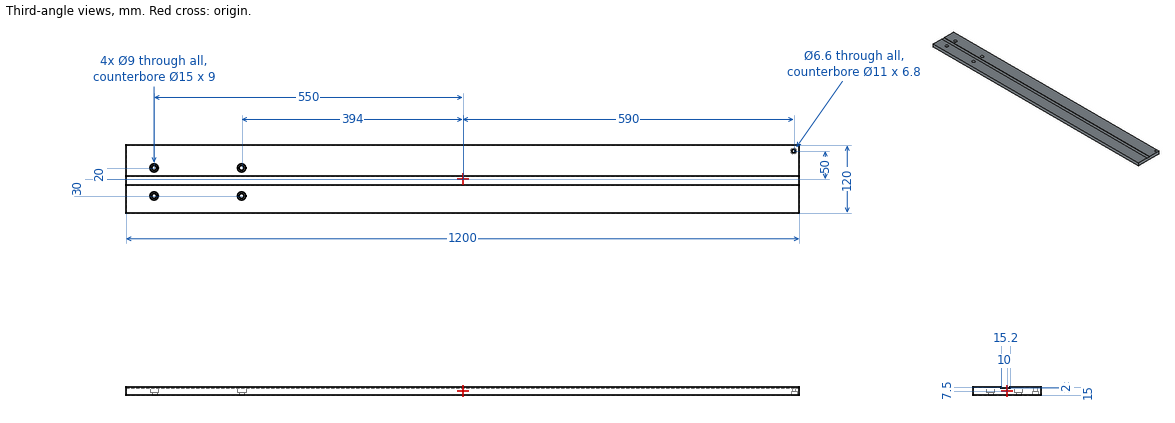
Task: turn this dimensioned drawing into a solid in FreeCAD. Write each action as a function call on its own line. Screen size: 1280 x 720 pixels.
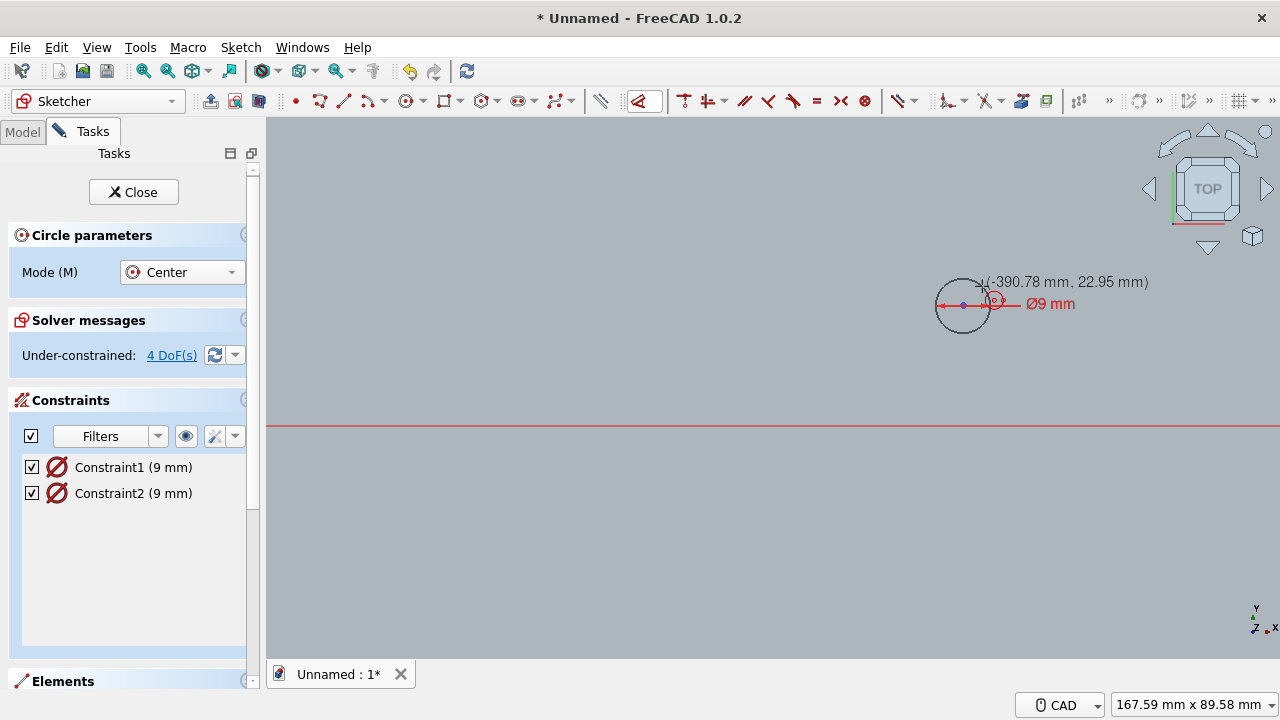
click(963, 607)
move(982, 588)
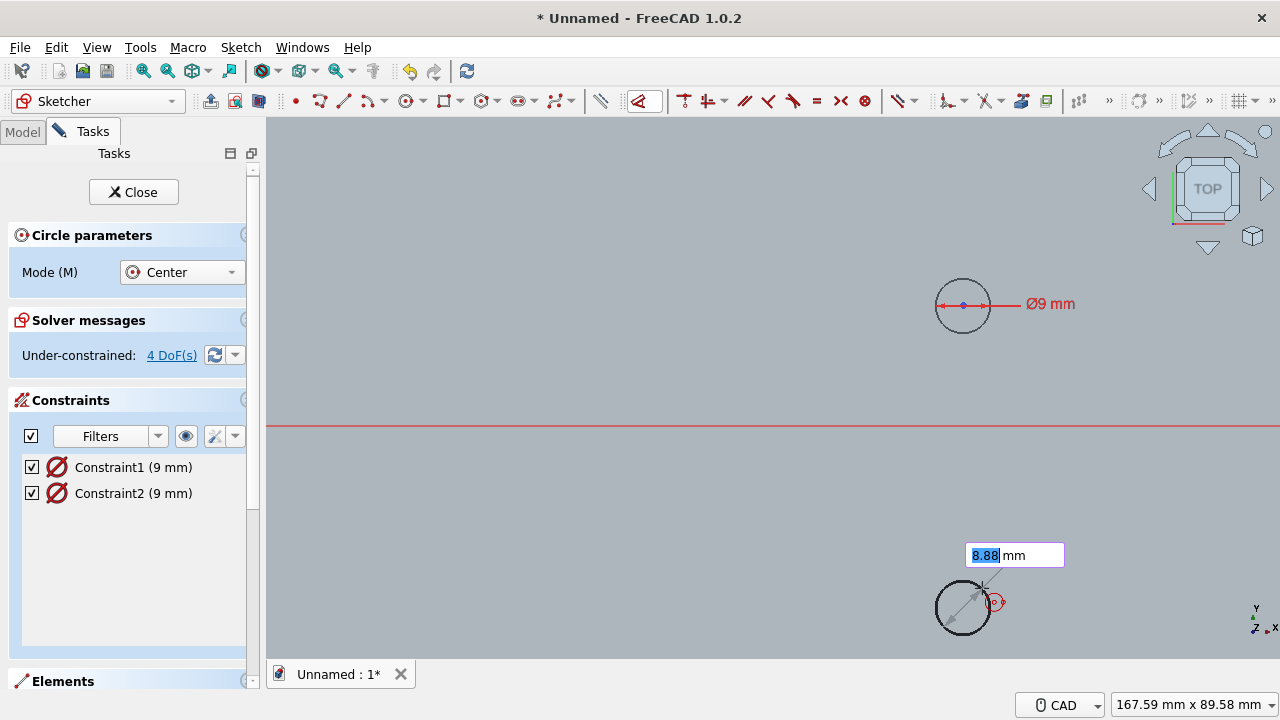
text(9)
key(Return)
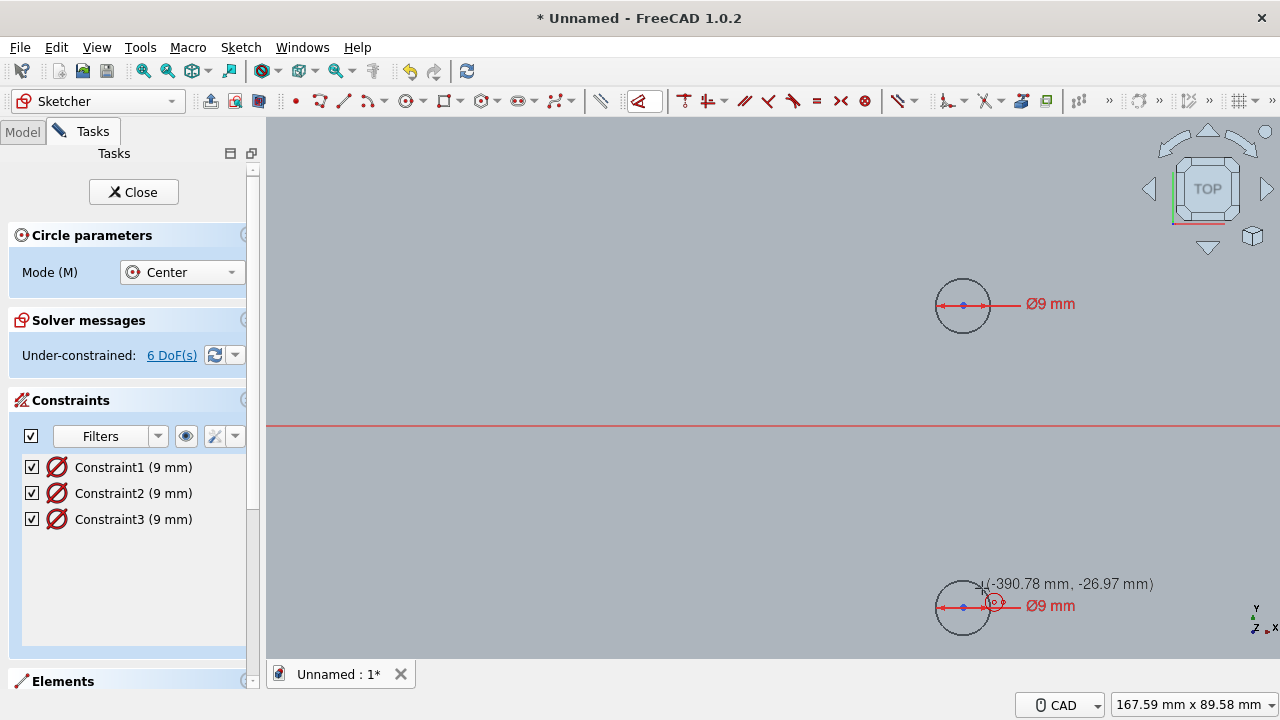
scroll(965, 305, down, 3)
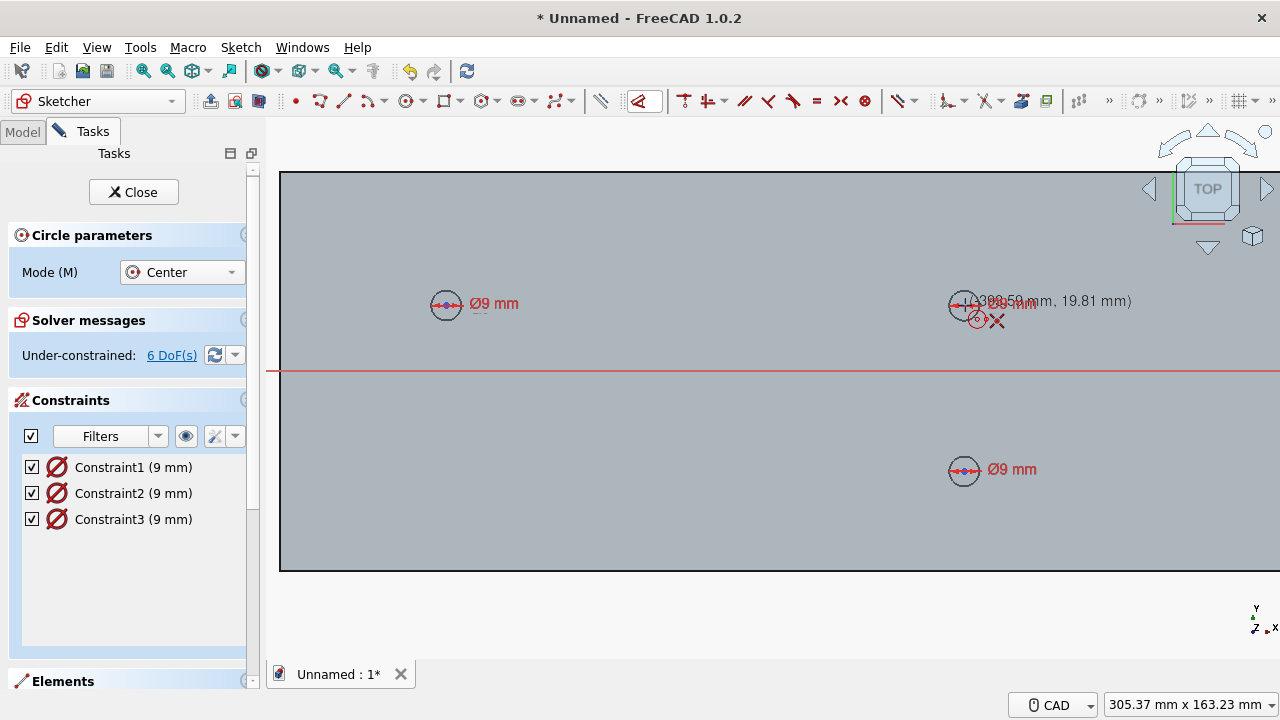
scroll(446, 471, up, 3)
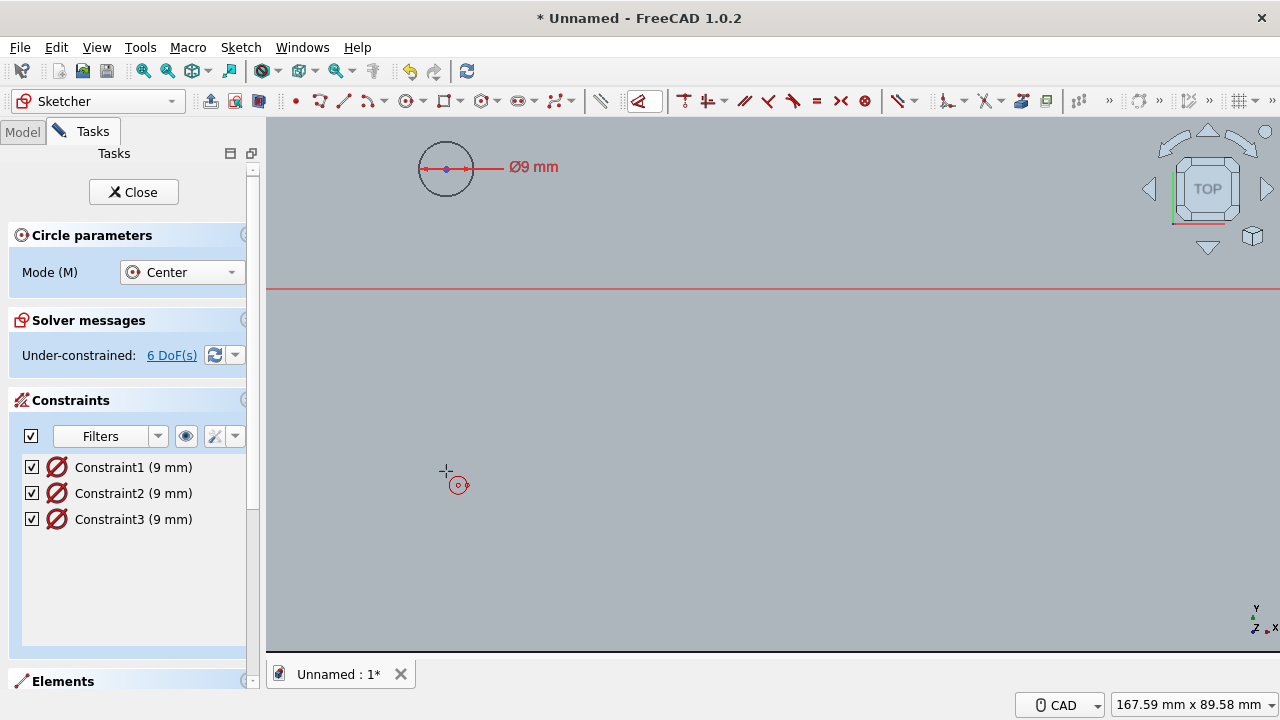
click(446, 471)
move(465, 451)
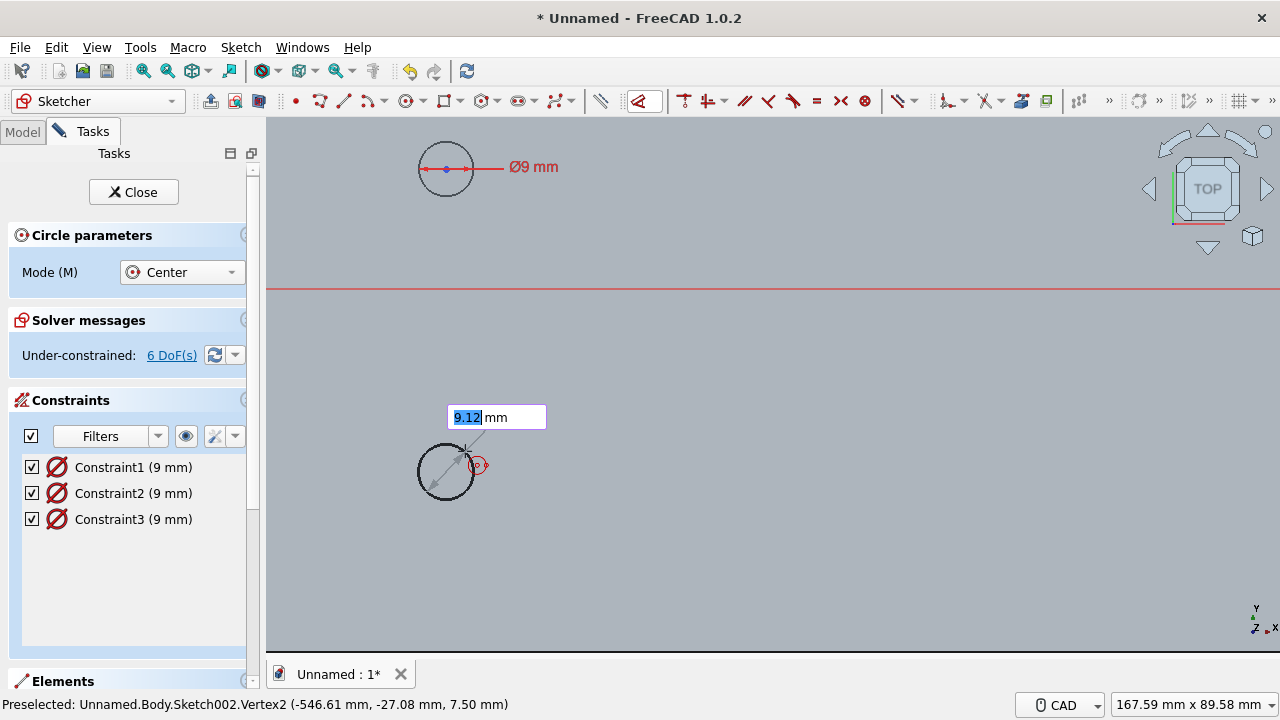
text(9)
key(Return)
key(Escape)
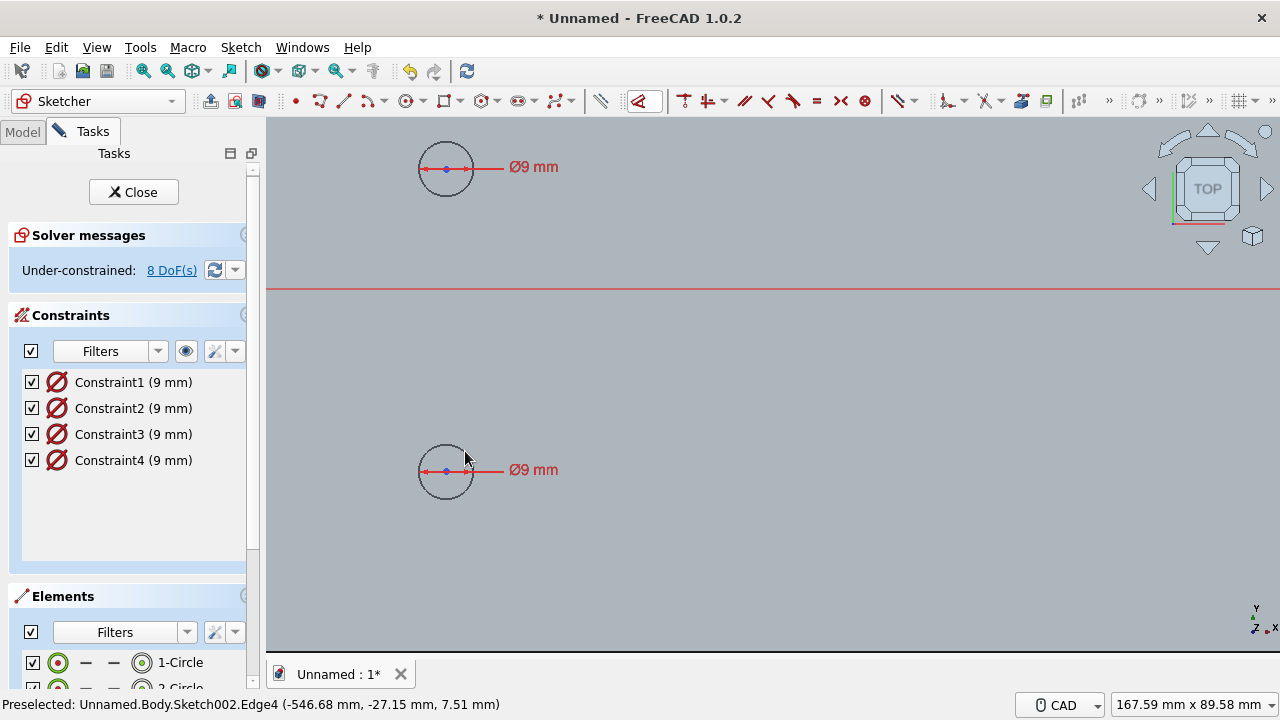
click(446, 169)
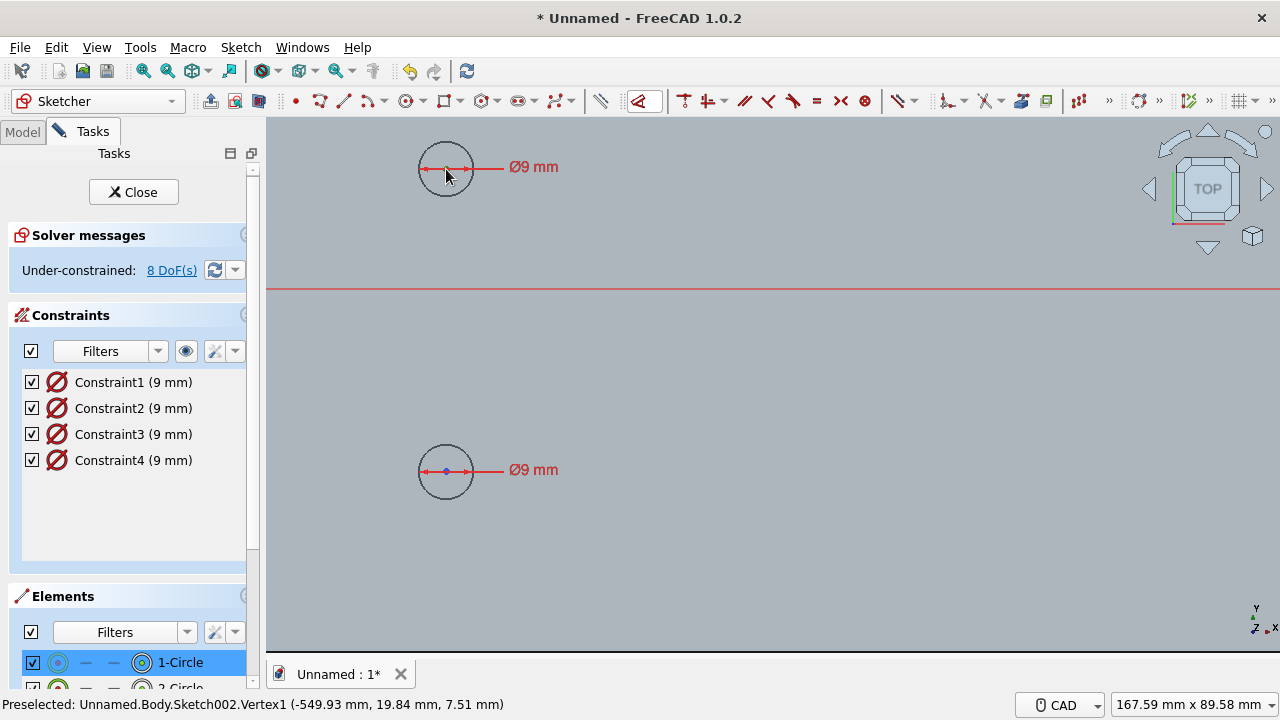
scroll(445, 471, down, 3)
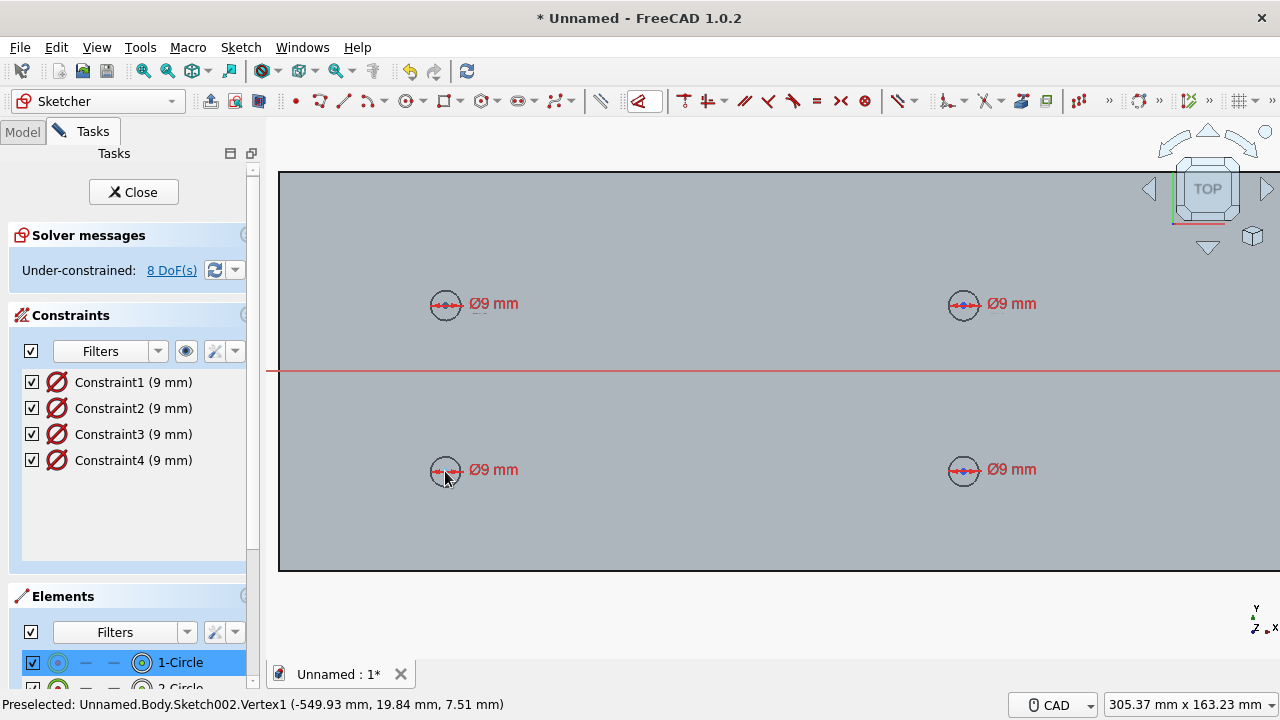
click(964, 306)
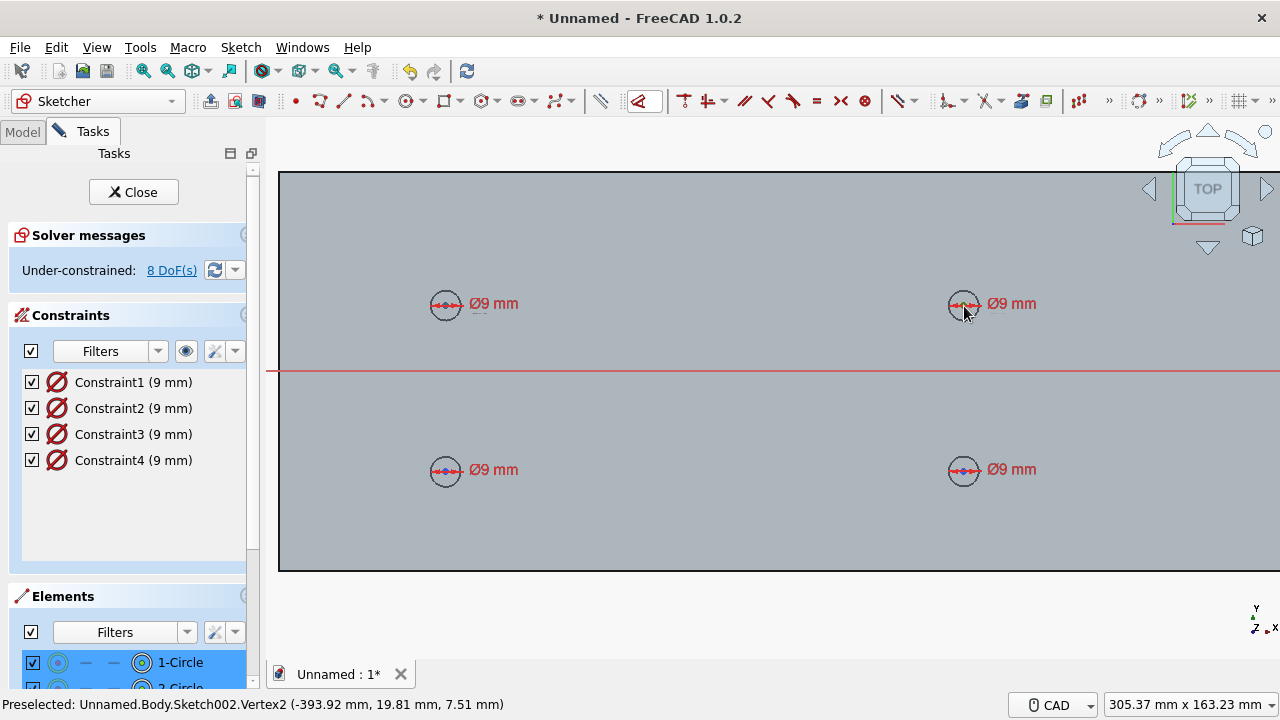
click(726, 102)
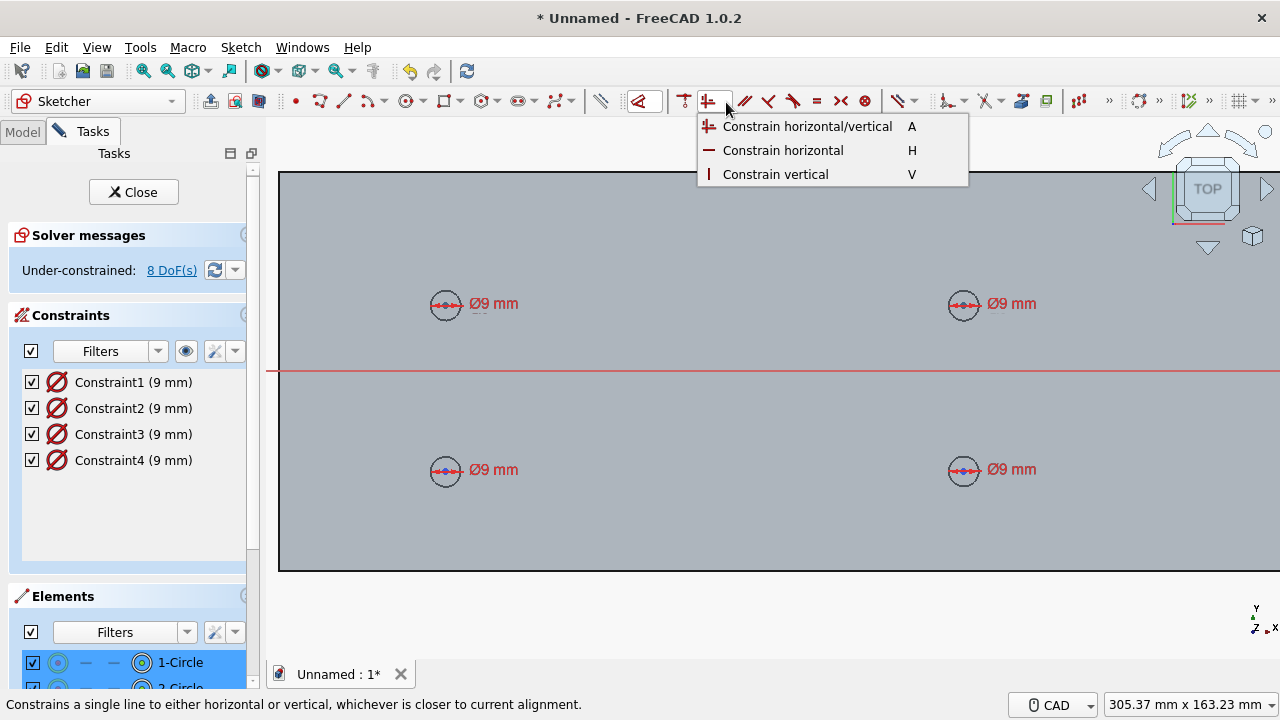
click(833, 150)